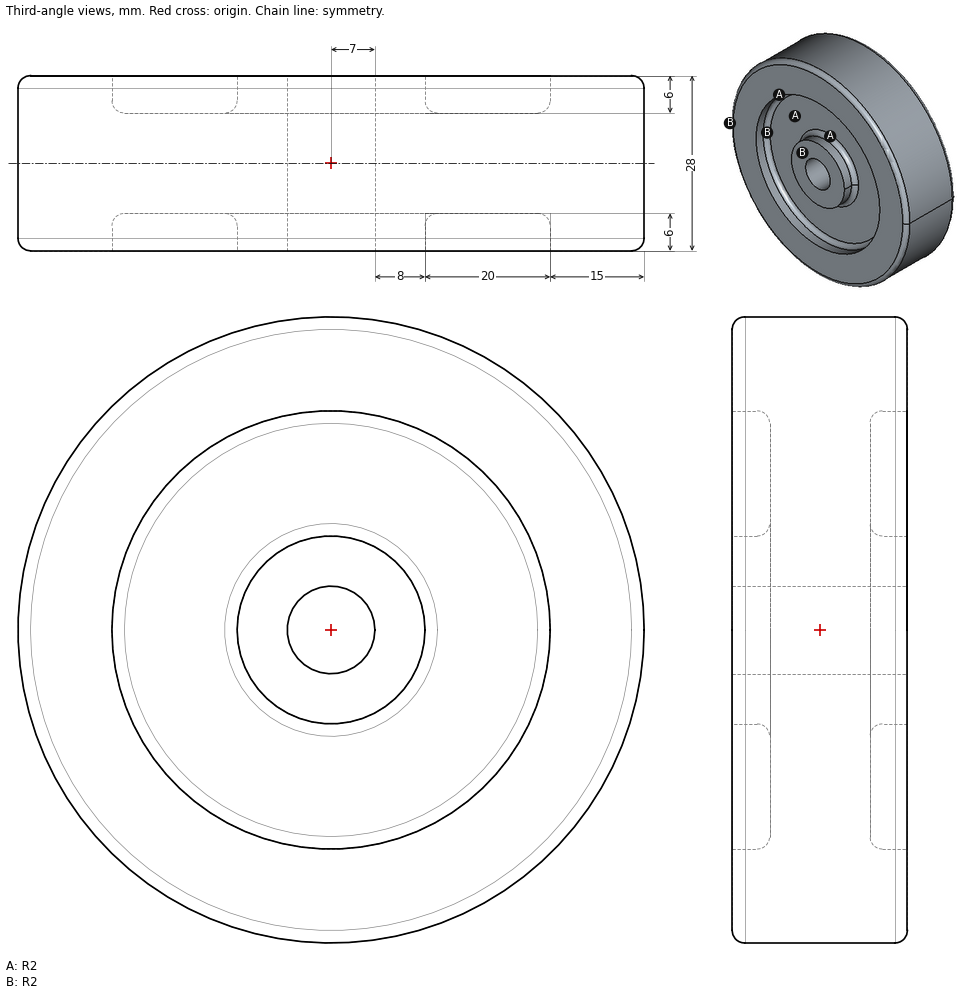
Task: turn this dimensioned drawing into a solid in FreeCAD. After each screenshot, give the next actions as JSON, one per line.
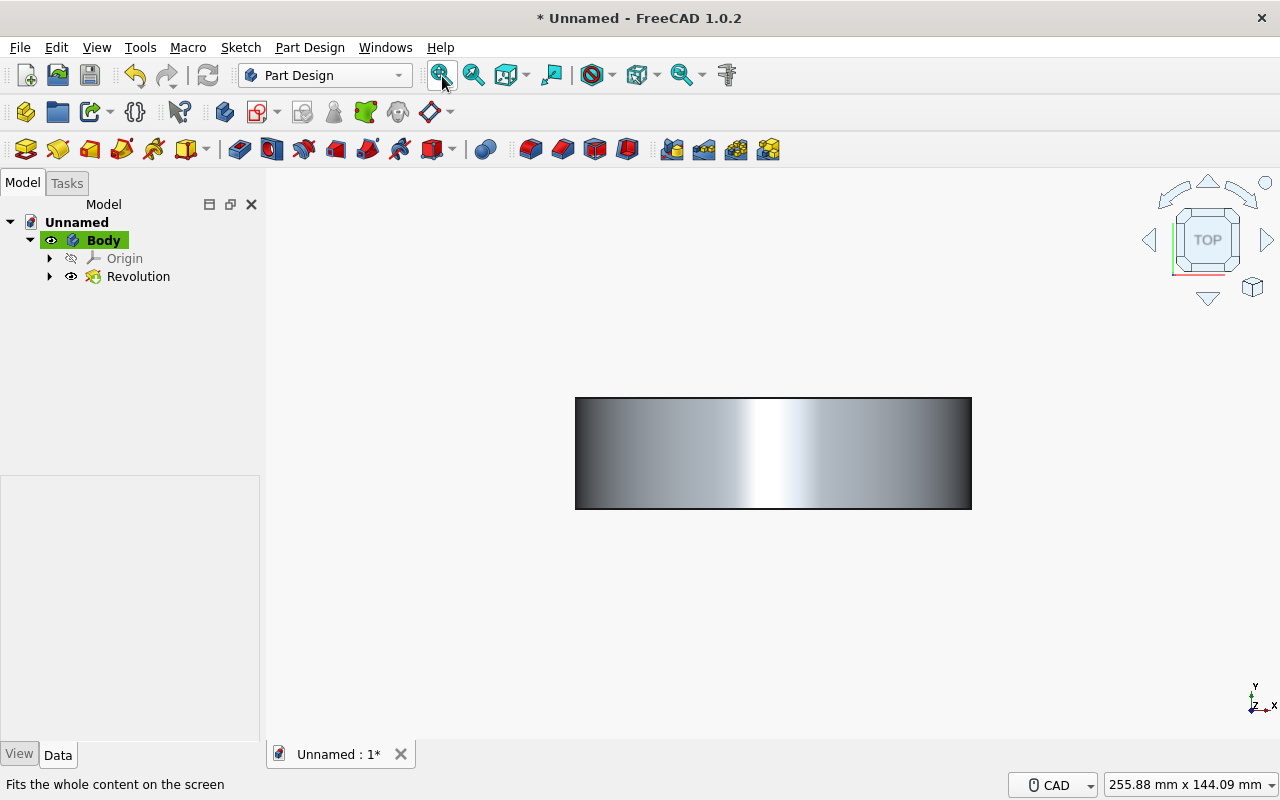
{"action": "left_click", "coordinate": [613, 397]}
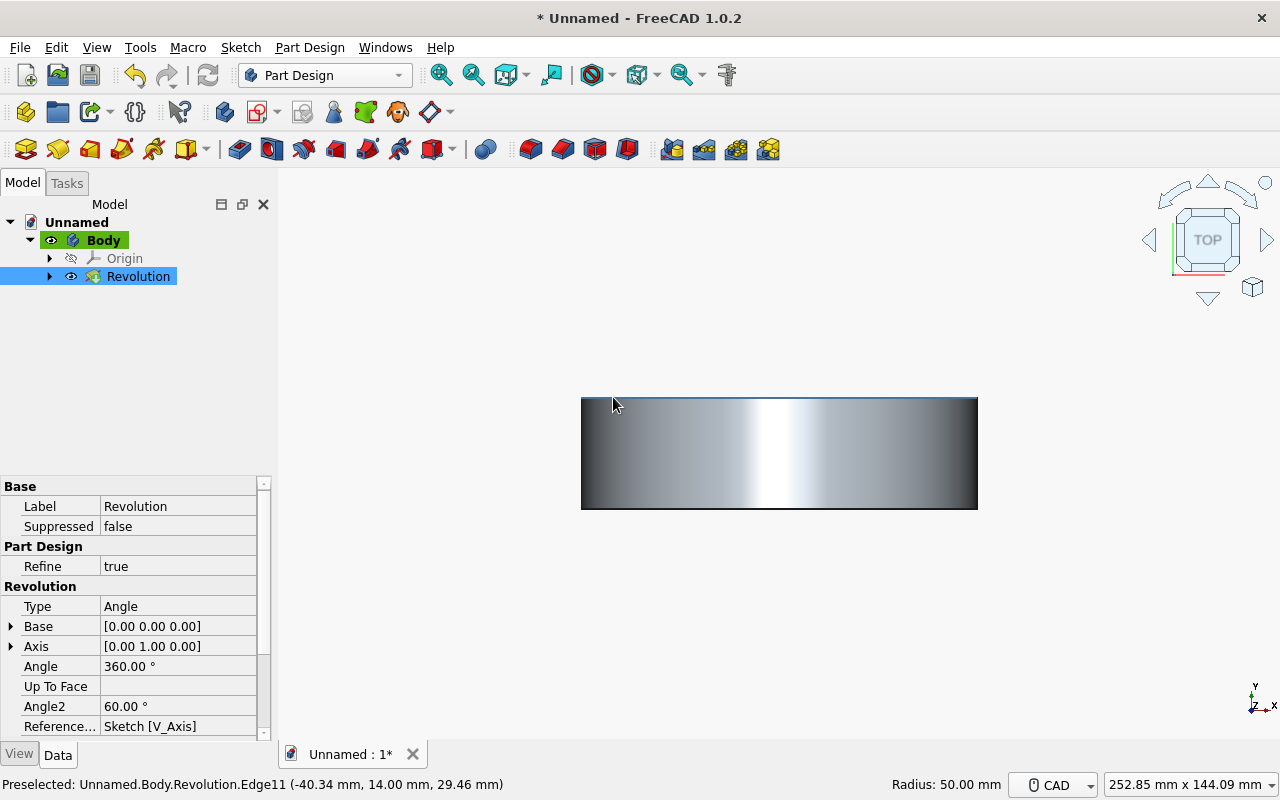
{"action": "key", "text": "1"}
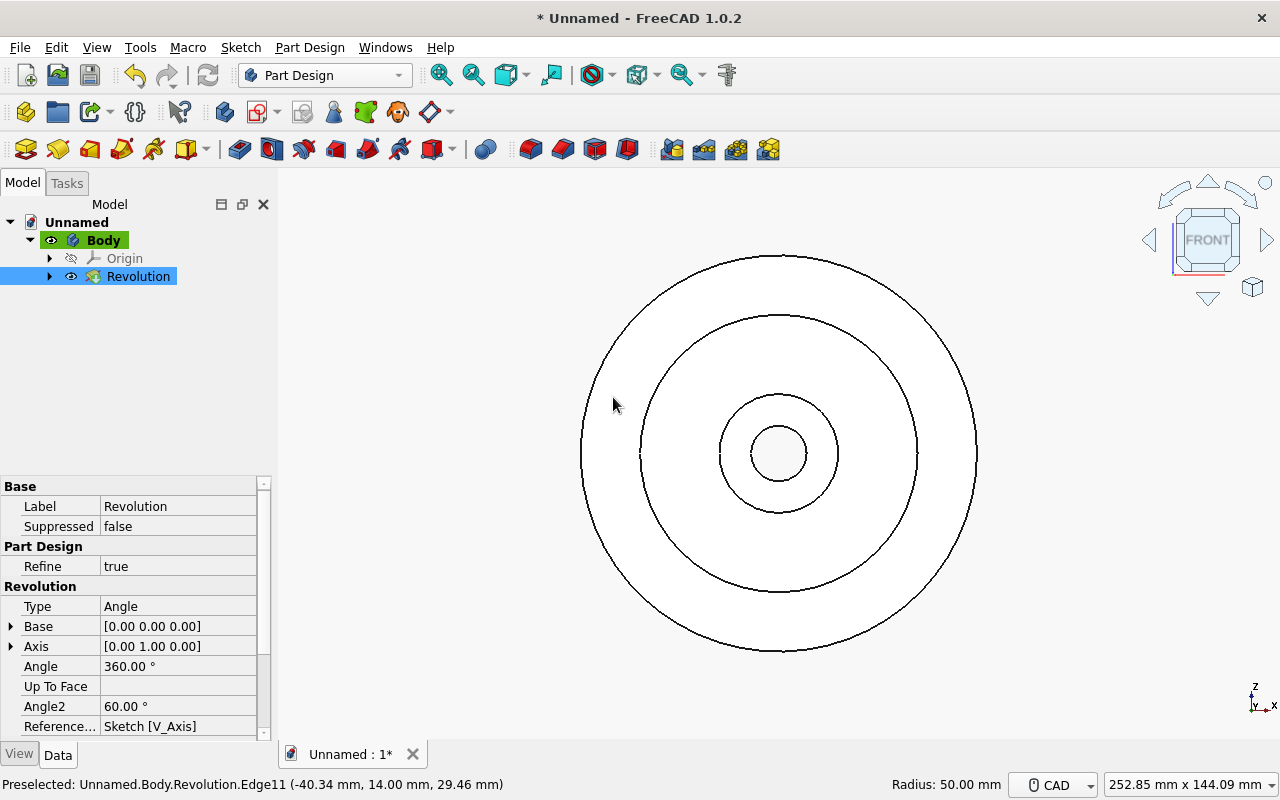
{"action": "key", "text": "3"}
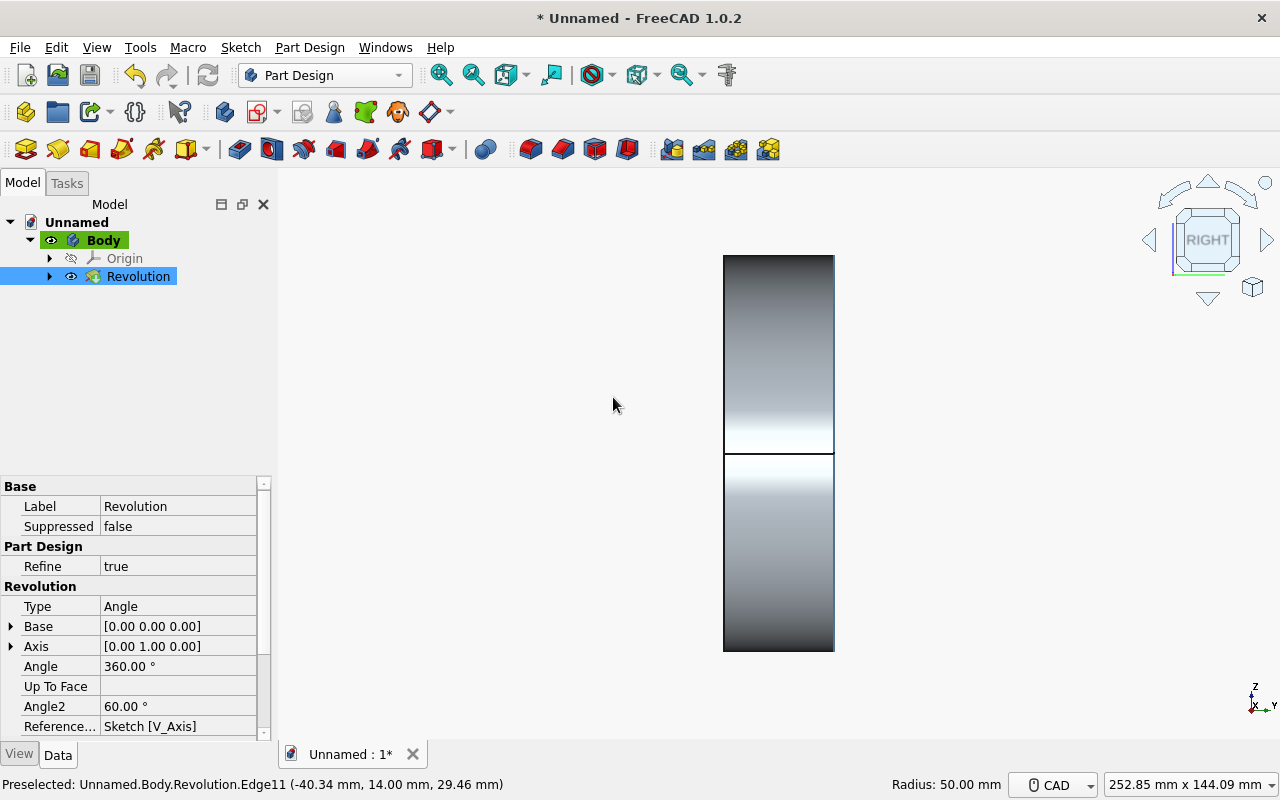
{"action": "key", "text": "5"}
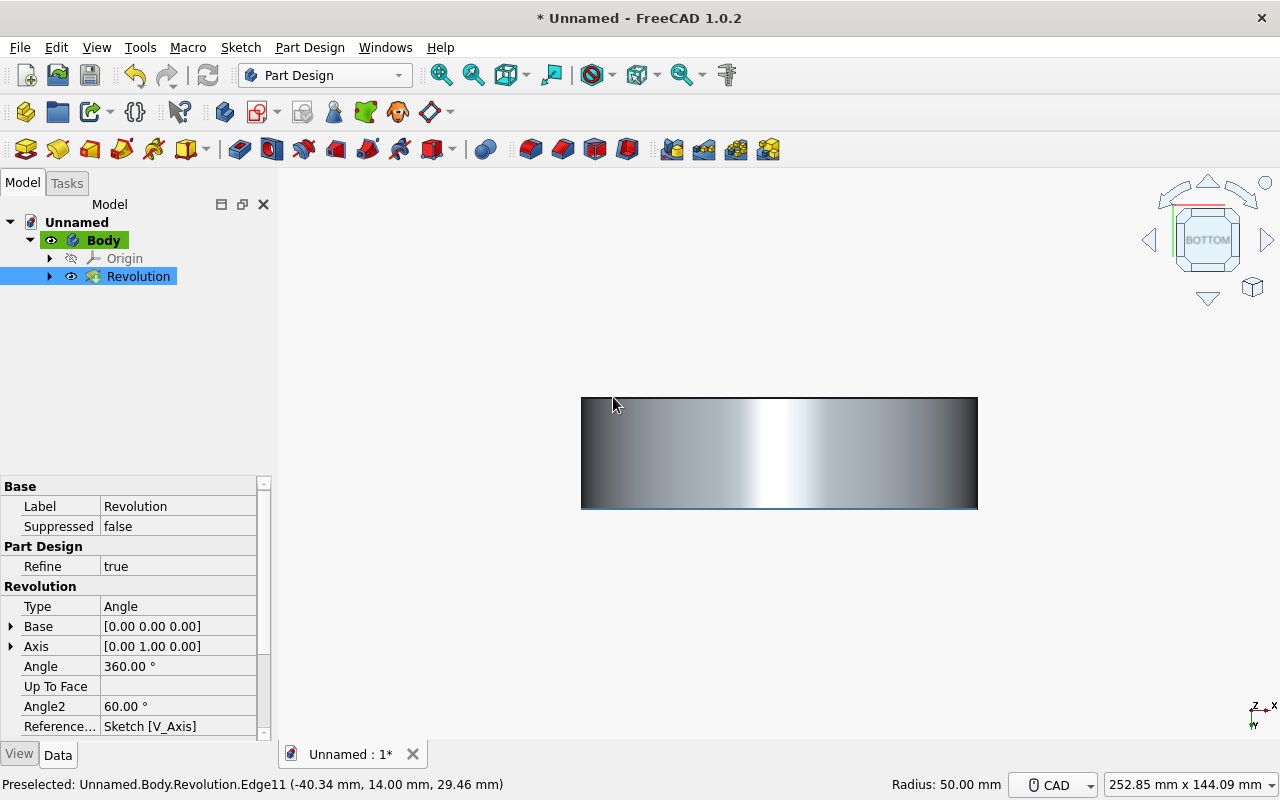
{"action": "left_click", "coordinate": [442, 76]}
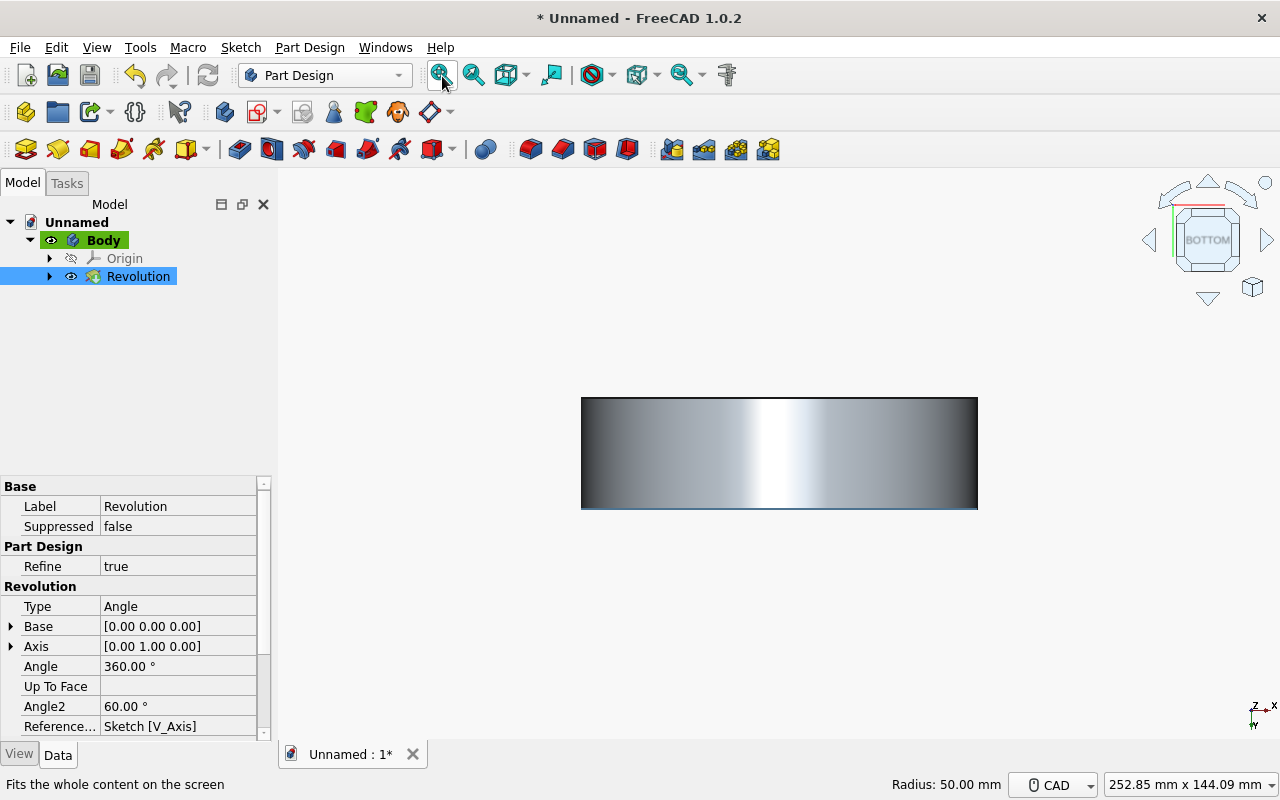
{"action": "key", "text": "4"}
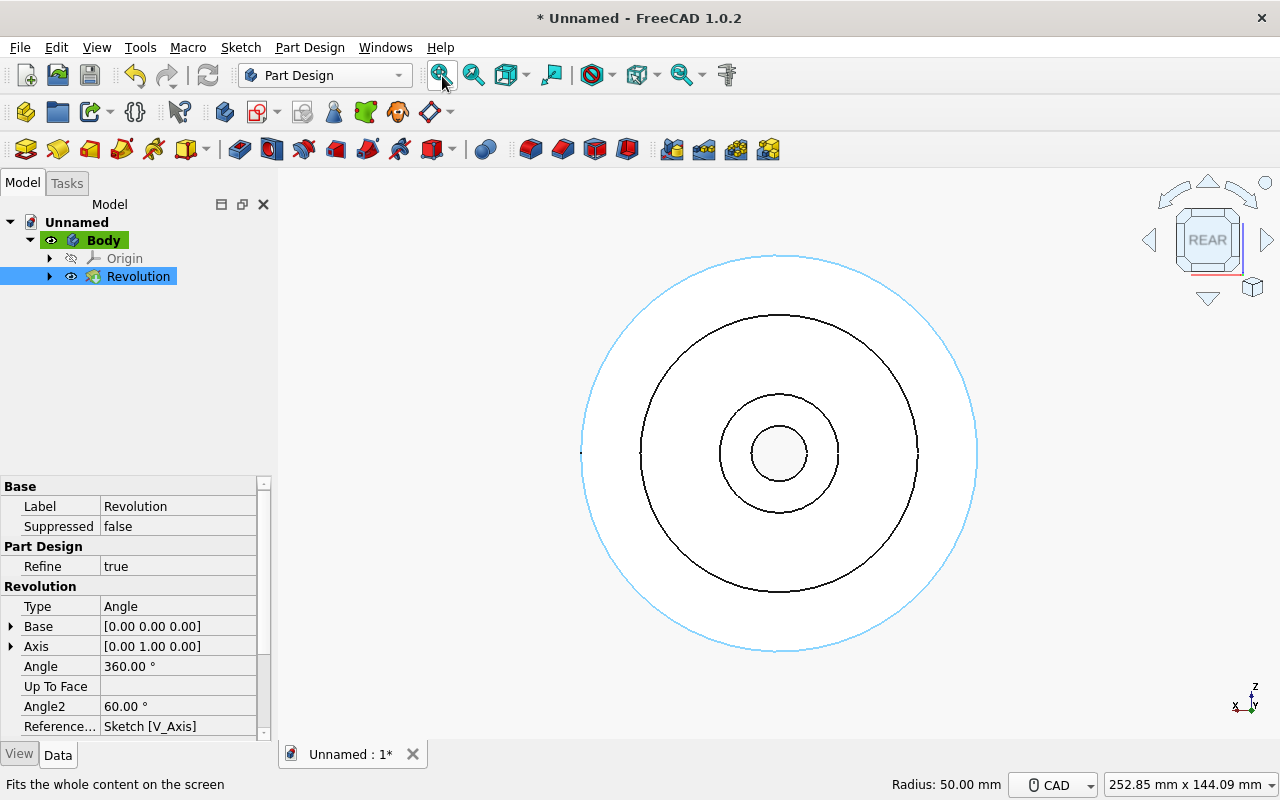
{"action": "key", "text": "6"}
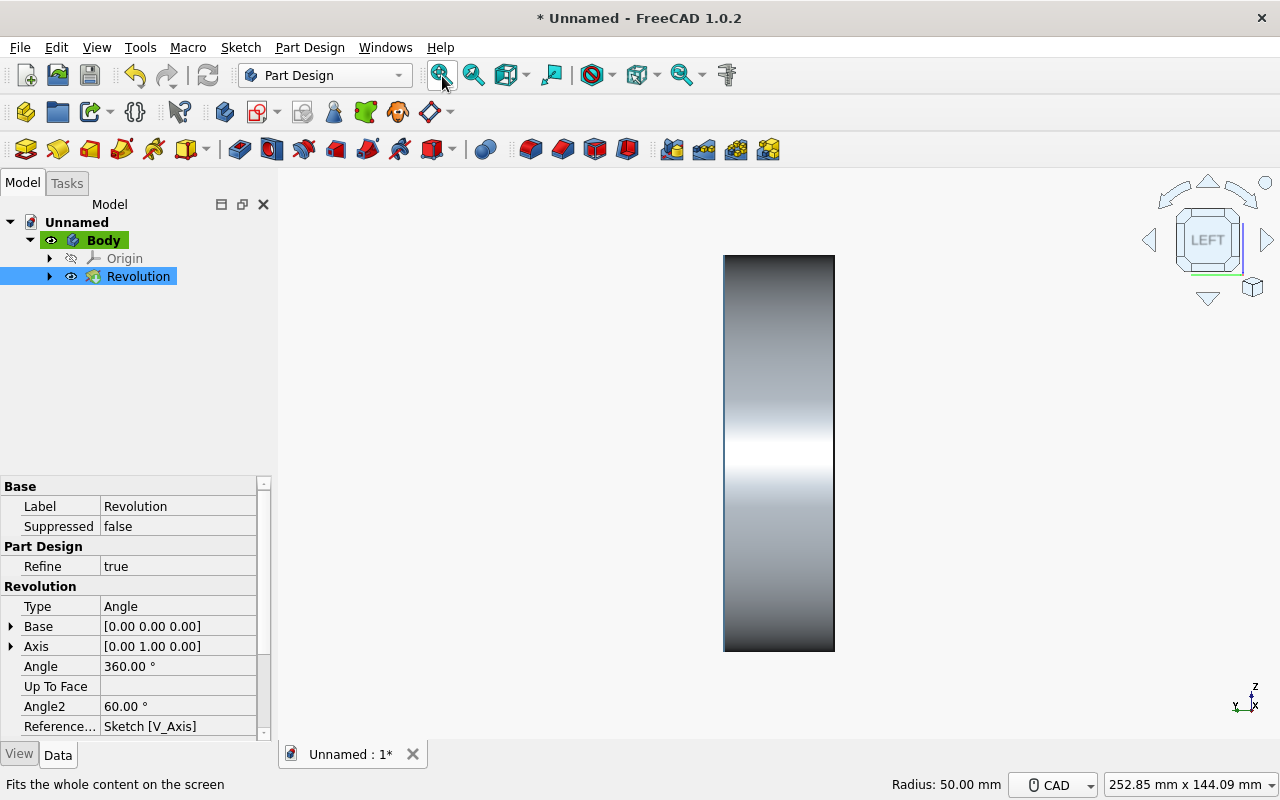
{"action": "key", "text": "v 3"}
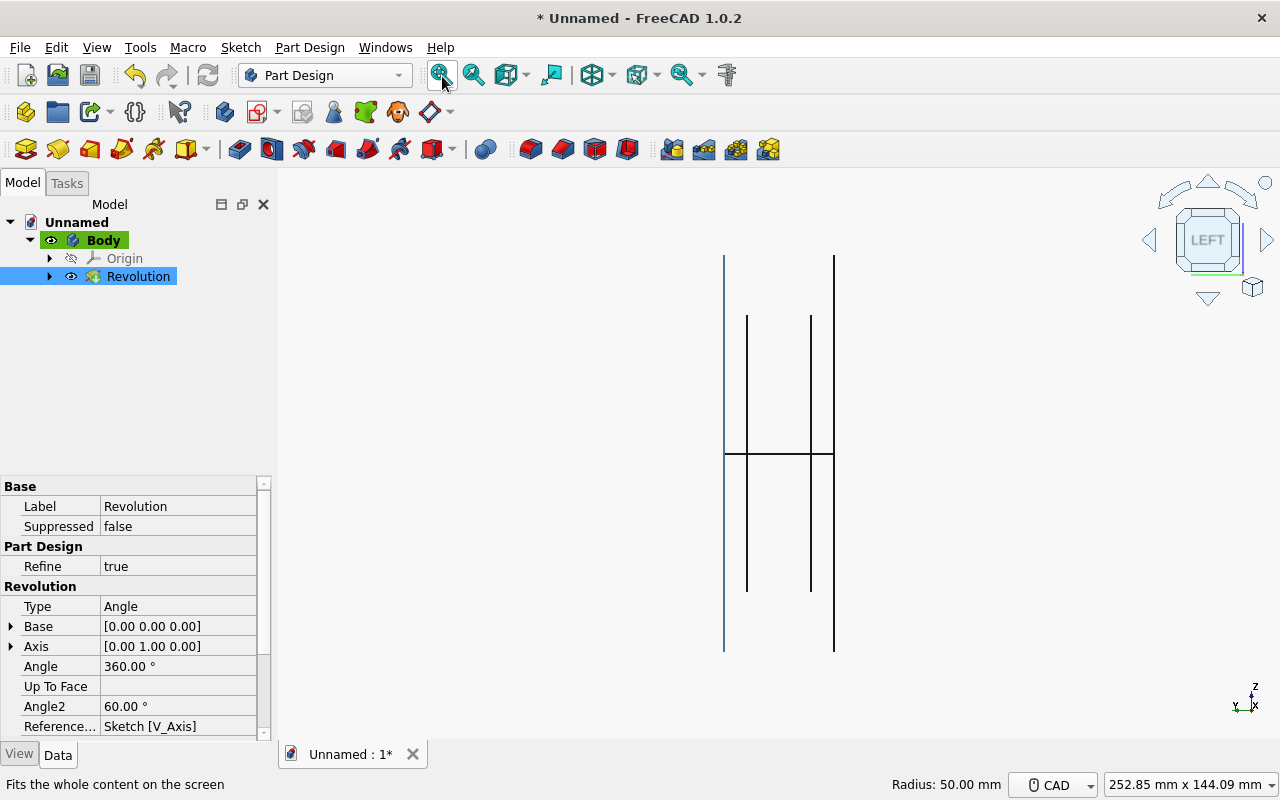
{"action": "key", "text": "0"}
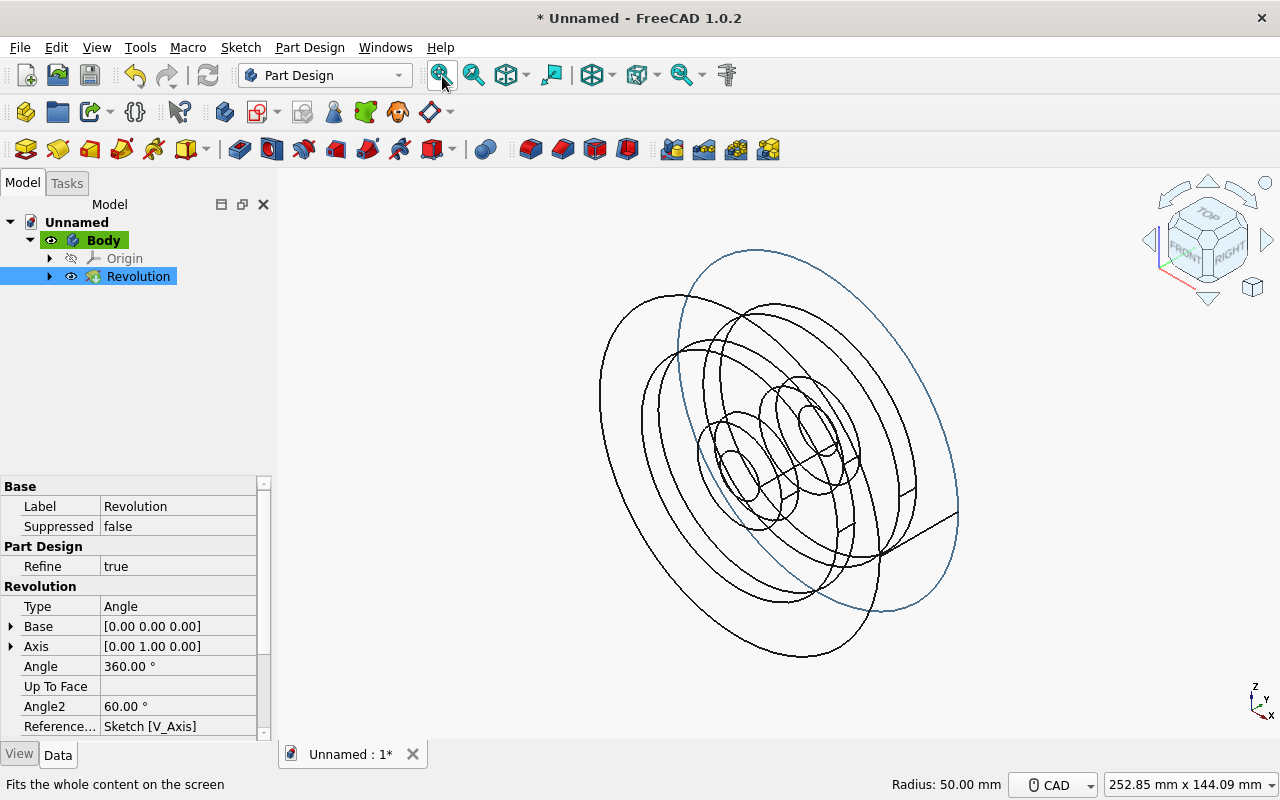
{"action": "left_click", "coordinate": [788, 386], "text": "ctrl"}